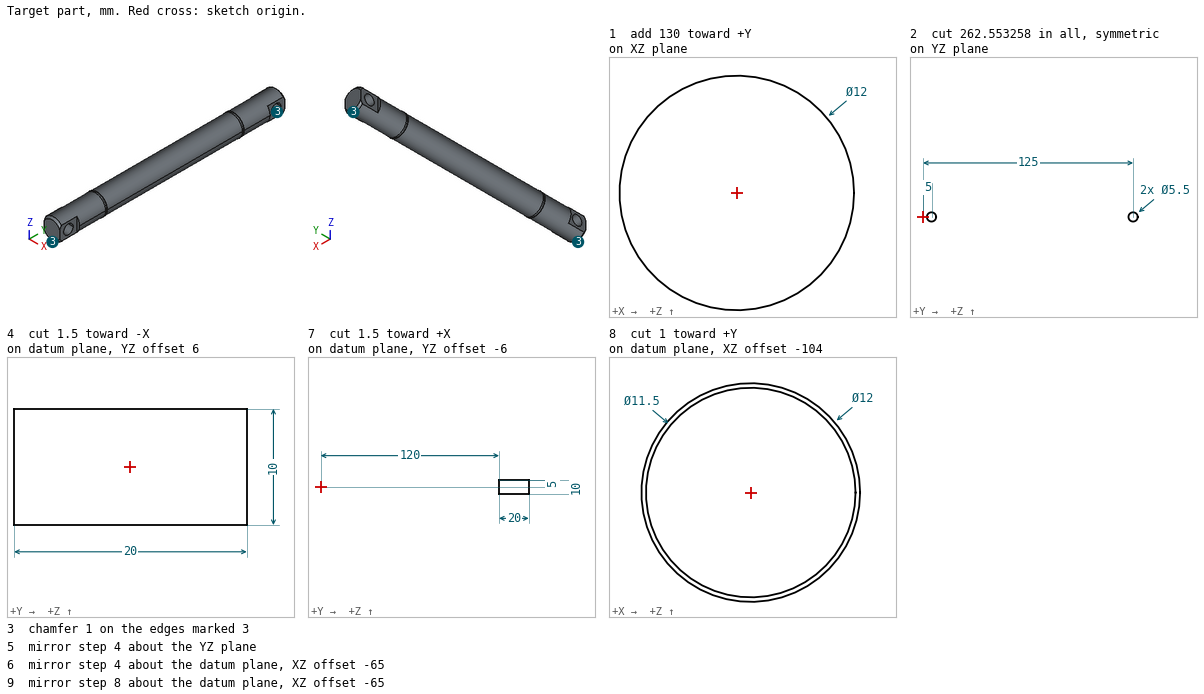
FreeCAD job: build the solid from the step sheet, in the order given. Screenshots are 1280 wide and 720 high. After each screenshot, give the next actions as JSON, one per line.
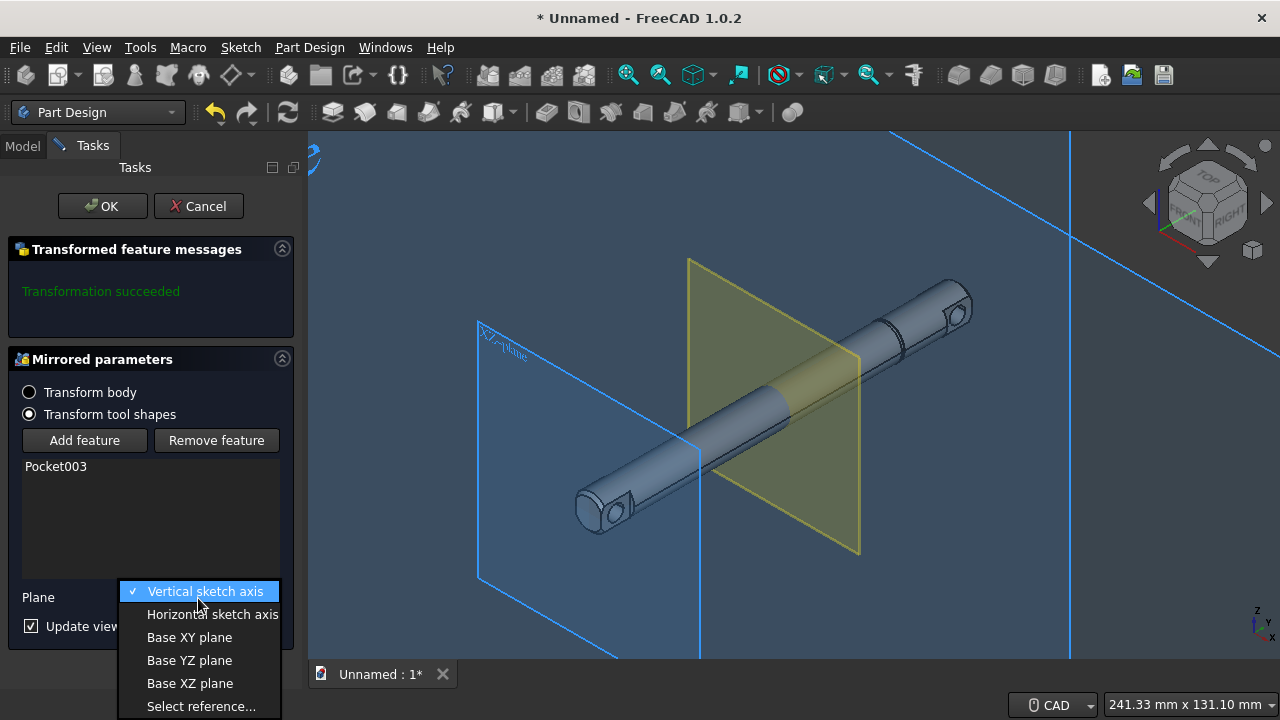
{"action": "left_click", "coordinate": [198, 706]}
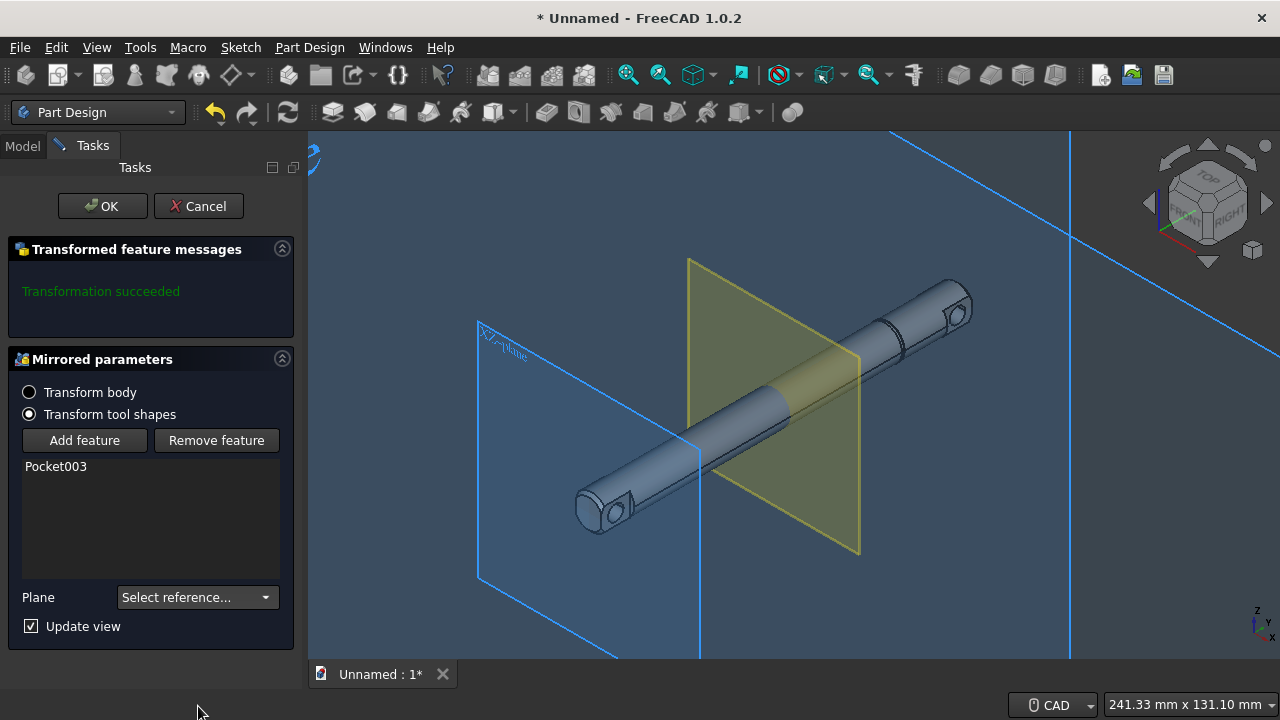
{"action": "left_click", "coordinate": [23, 145]}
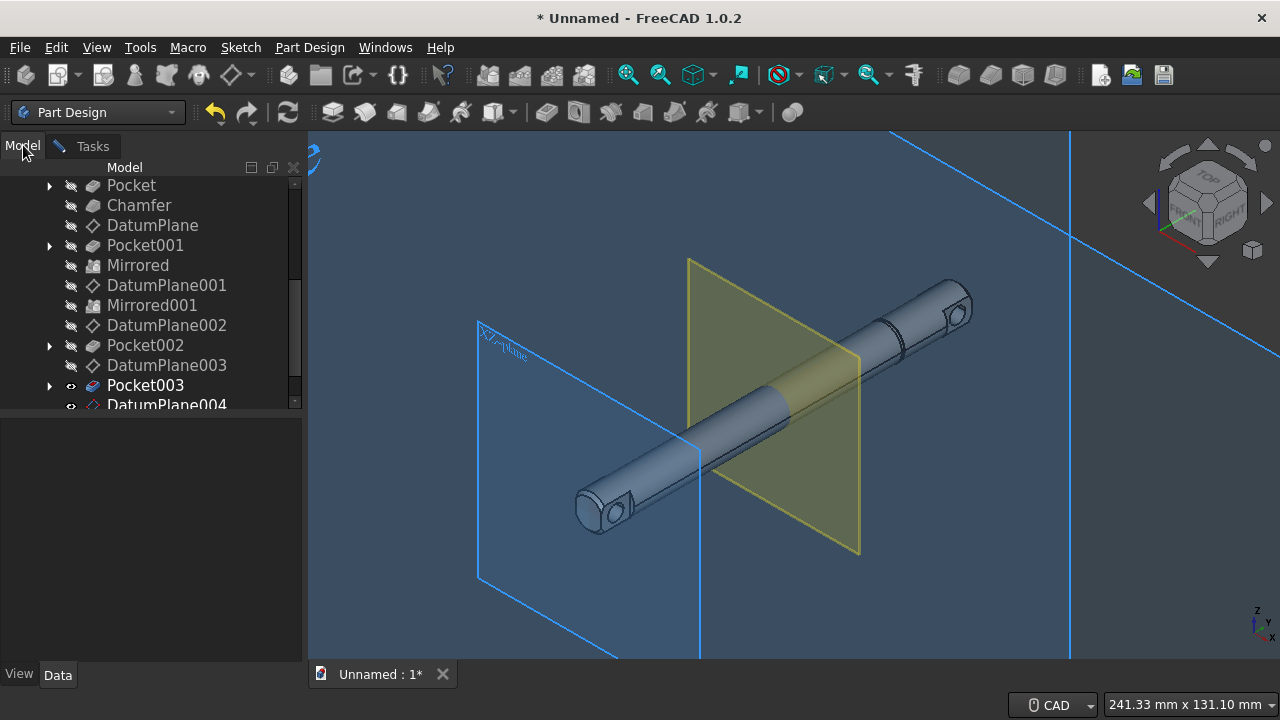
{"action": "left_click", "coordinate": [116, 406]}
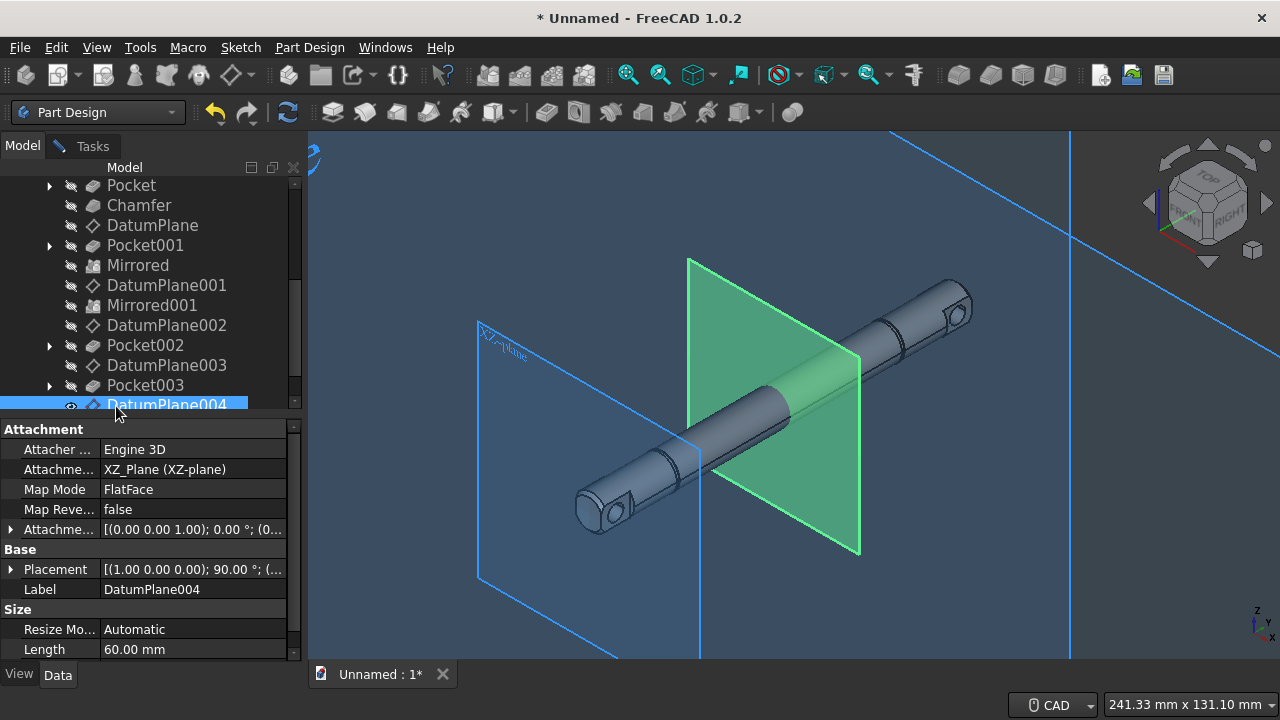
{"action": "left_click", "coordinate": [84, 145]}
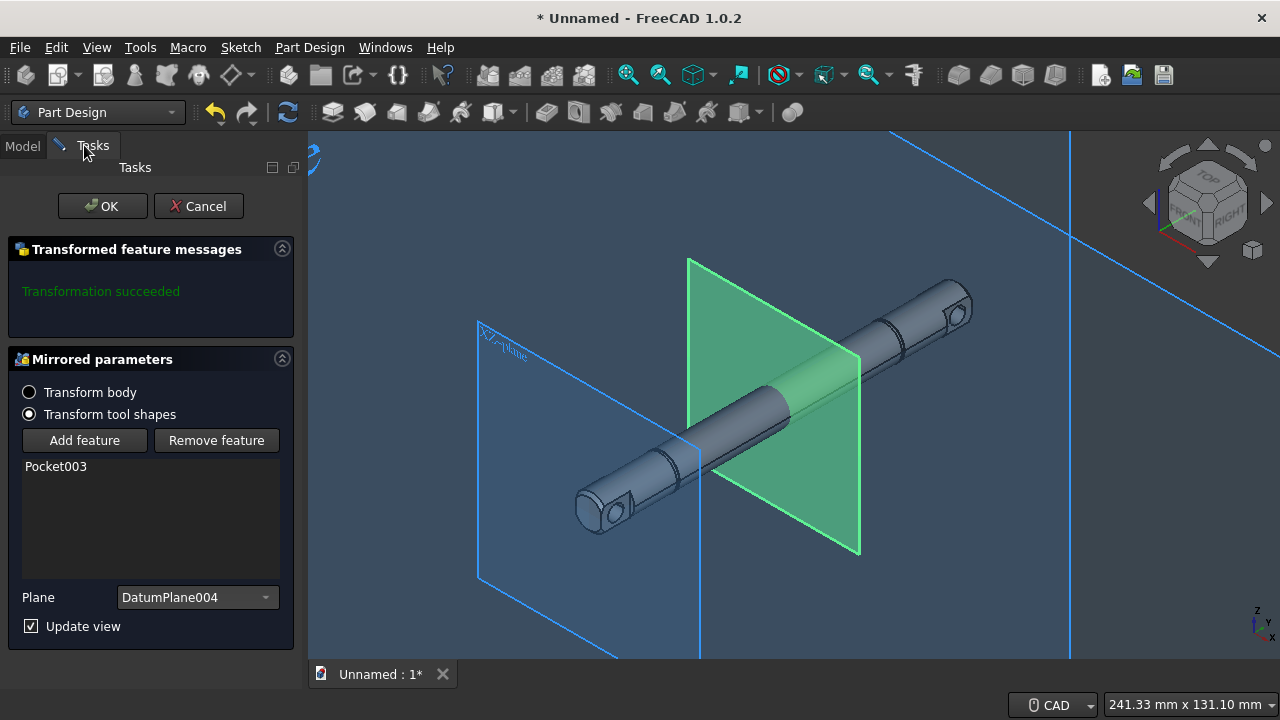
{"action": "left_click", "coordinate": [103, 206]}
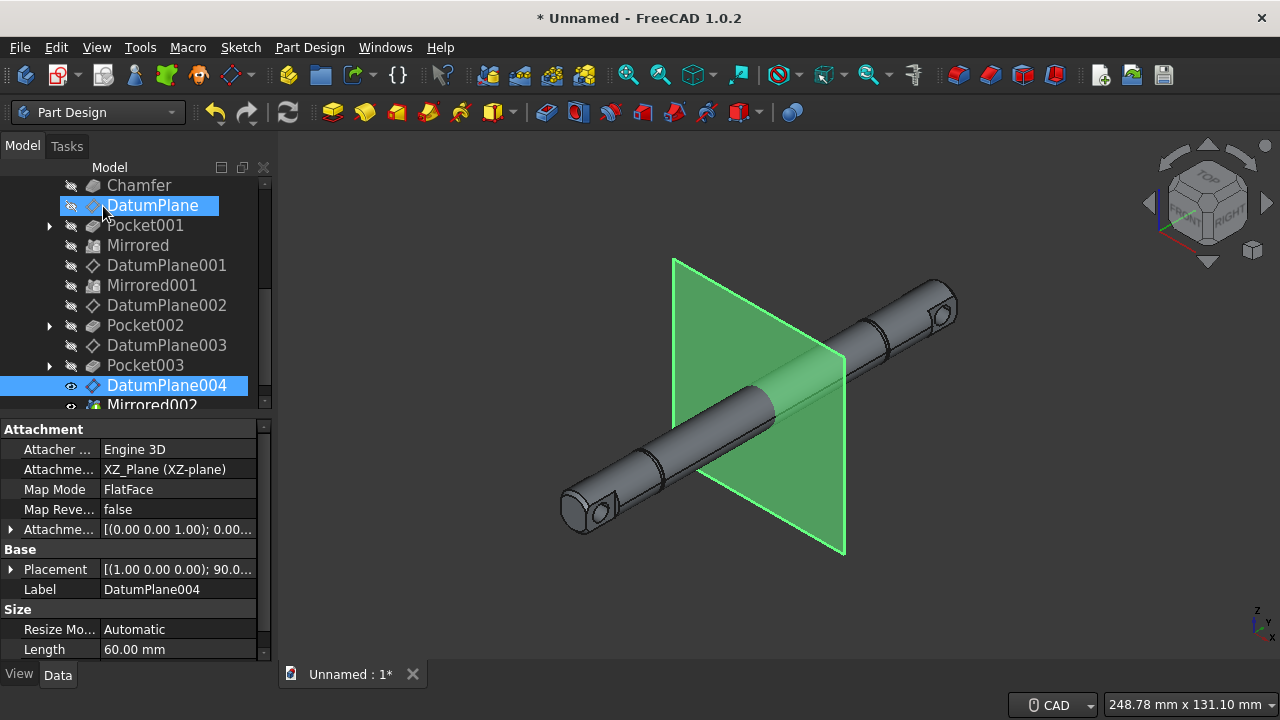
{"action": "left_click", "coordinate": [116, 386]}
{"action": "key", "text": "space"}